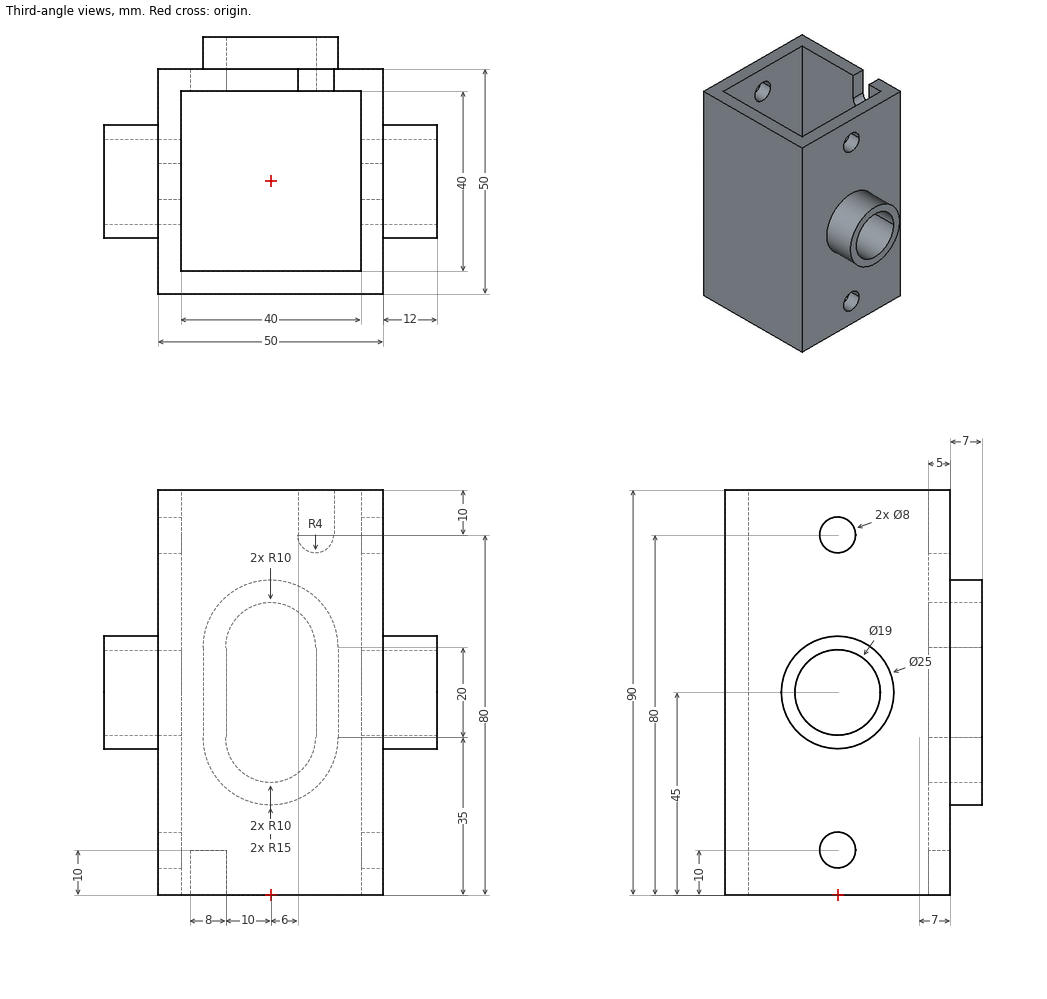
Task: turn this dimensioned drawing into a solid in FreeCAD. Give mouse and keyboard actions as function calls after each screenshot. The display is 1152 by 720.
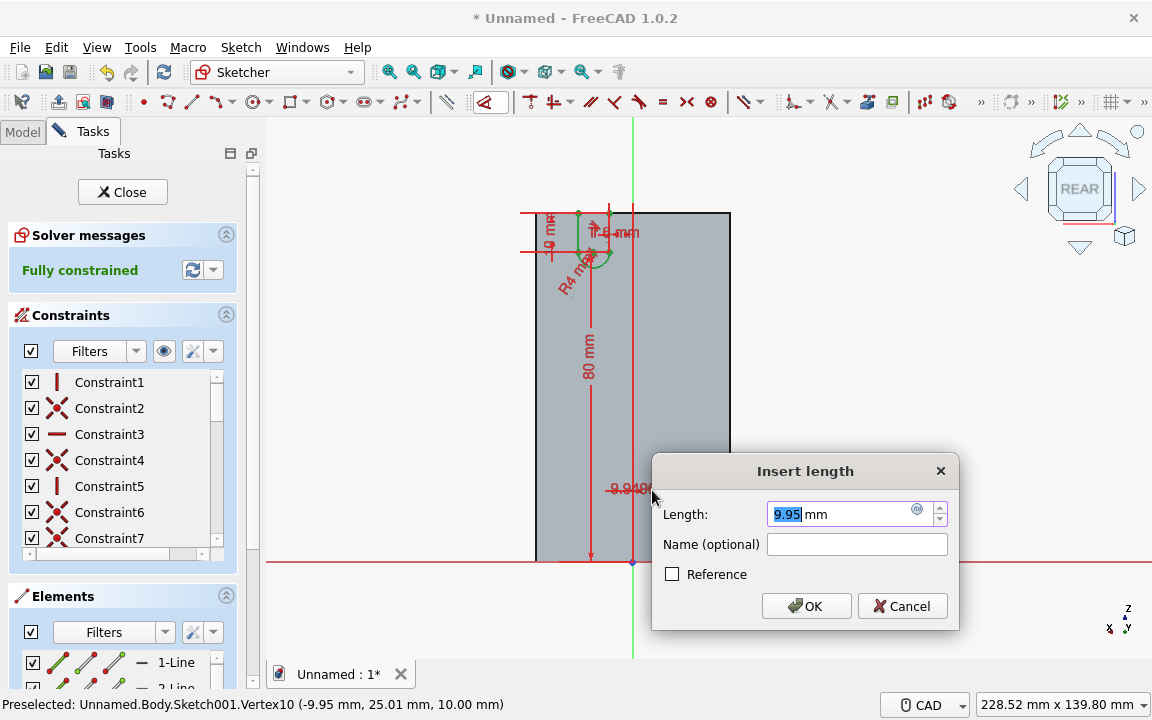
text(10)
key(Return)
key(Escape)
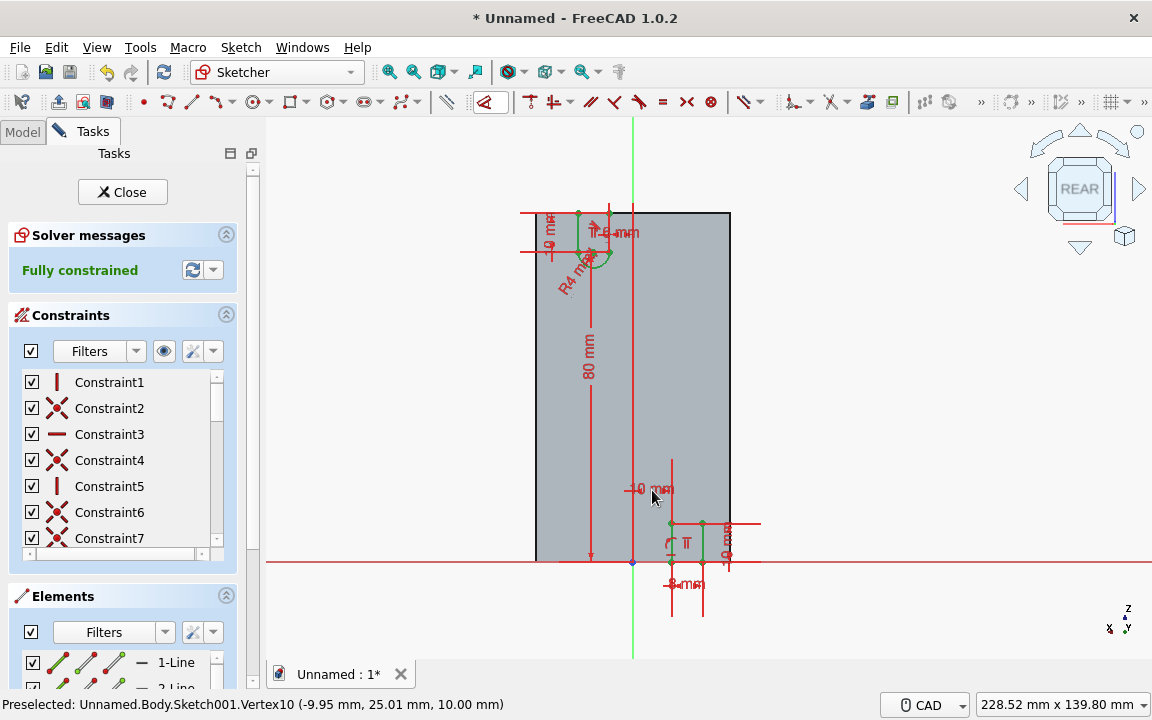
click(123, 192)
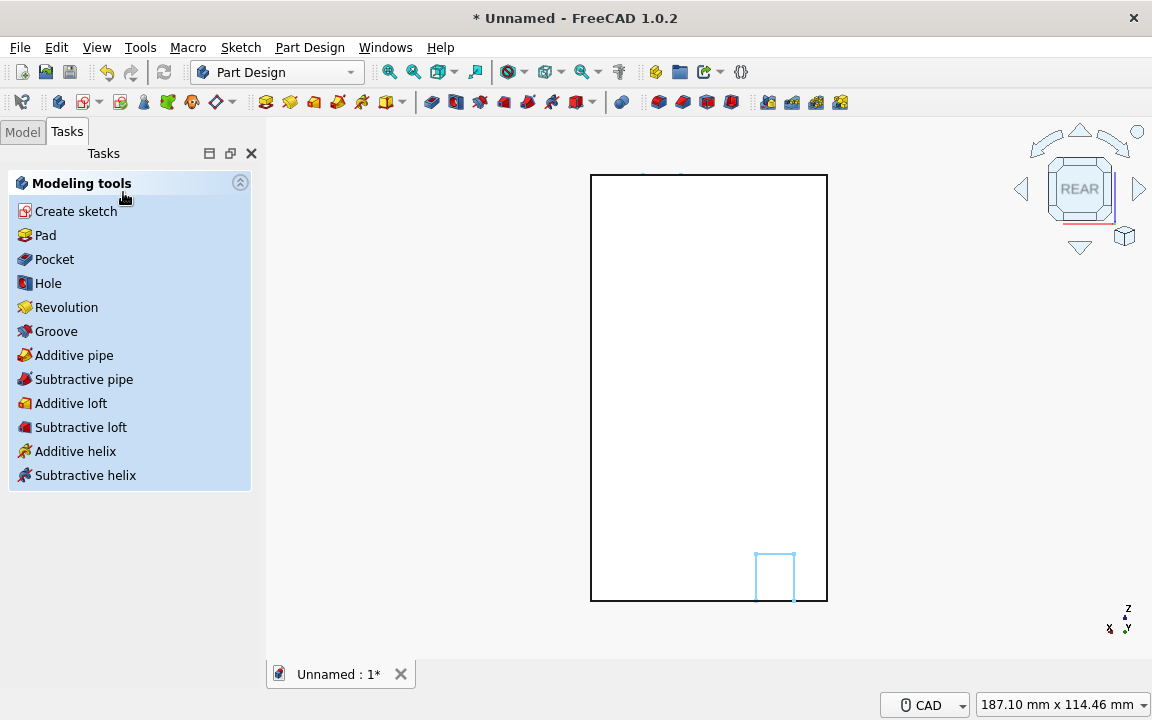
click(432, 102)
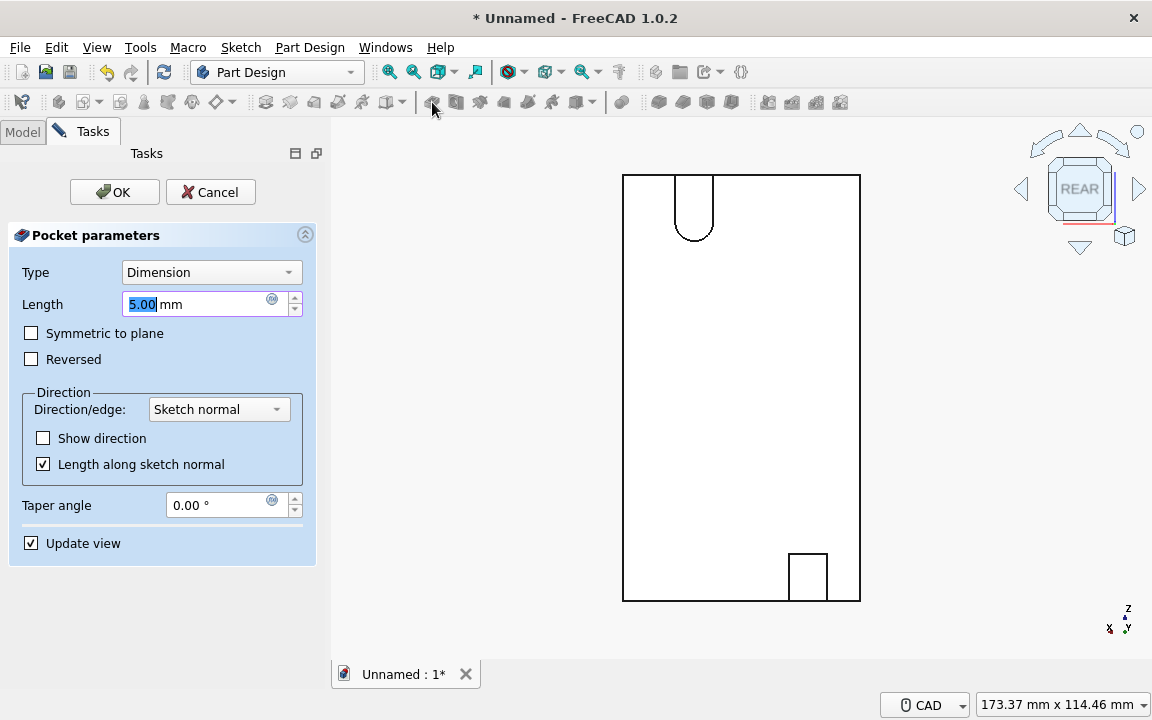
text(5)
key(Tab)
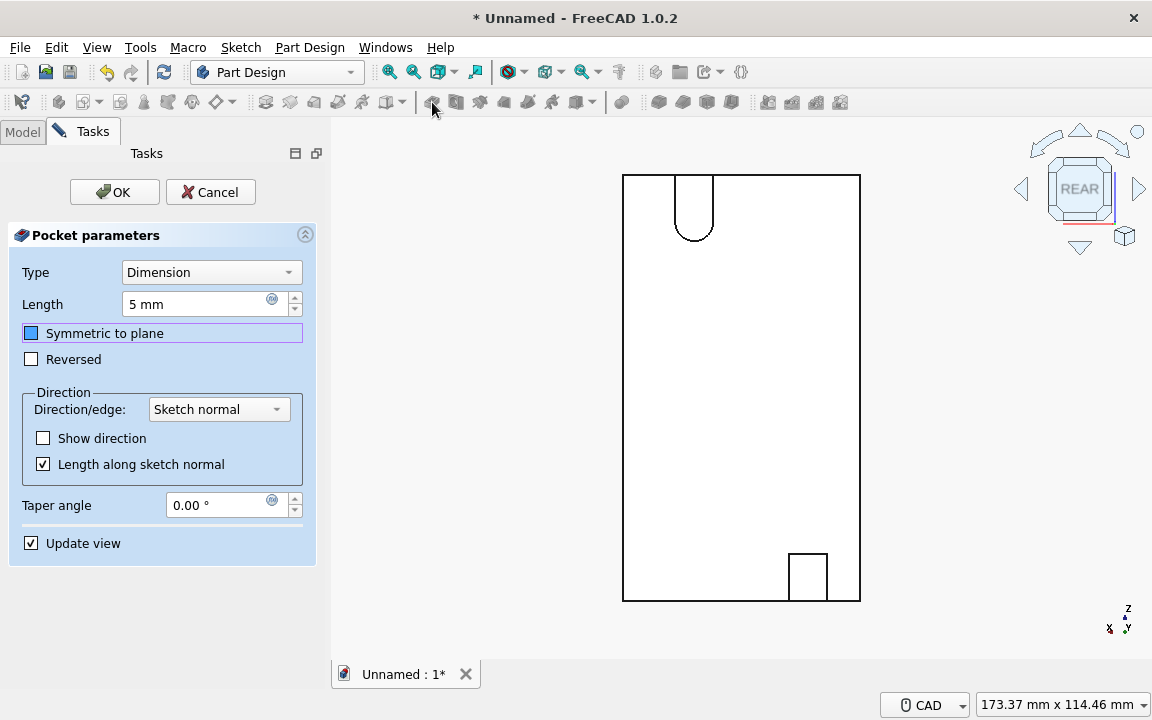
click(115, 192)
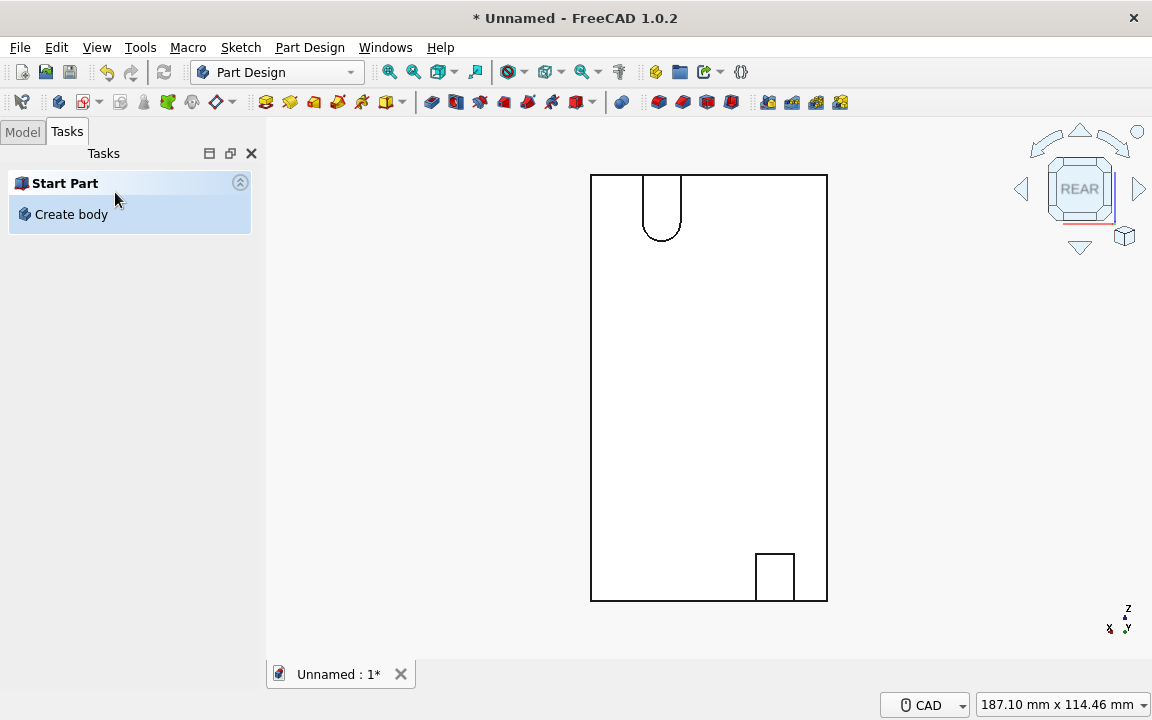
click(709, 387)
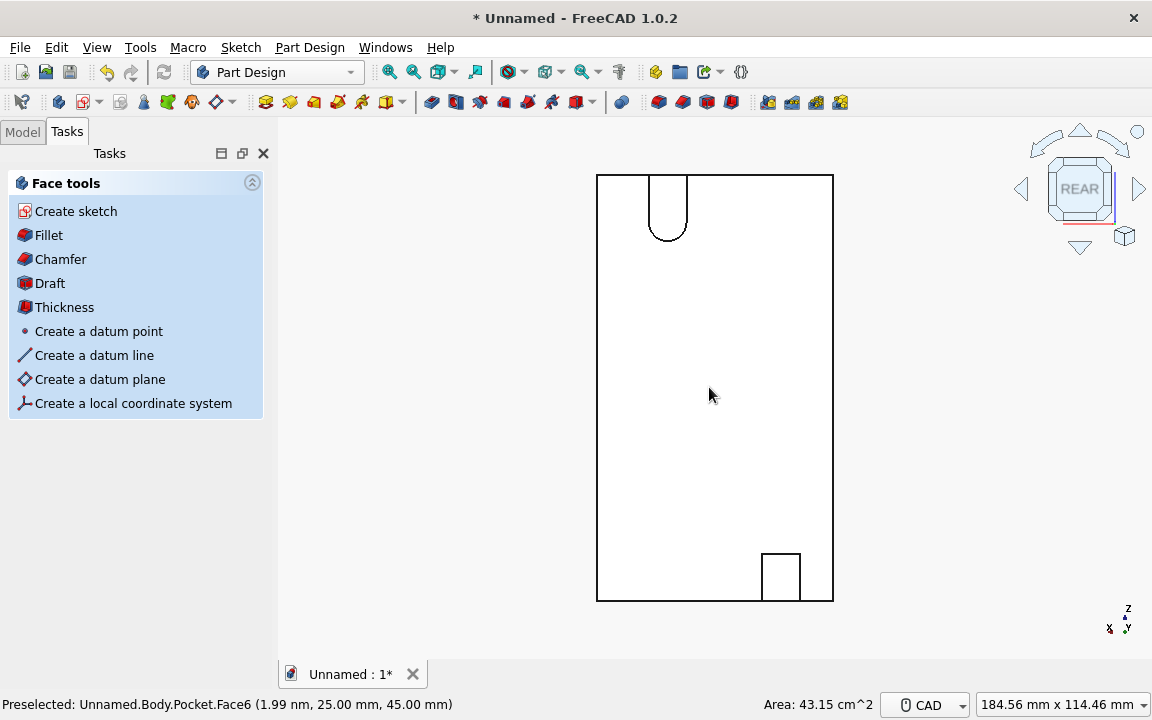
click(84, 102)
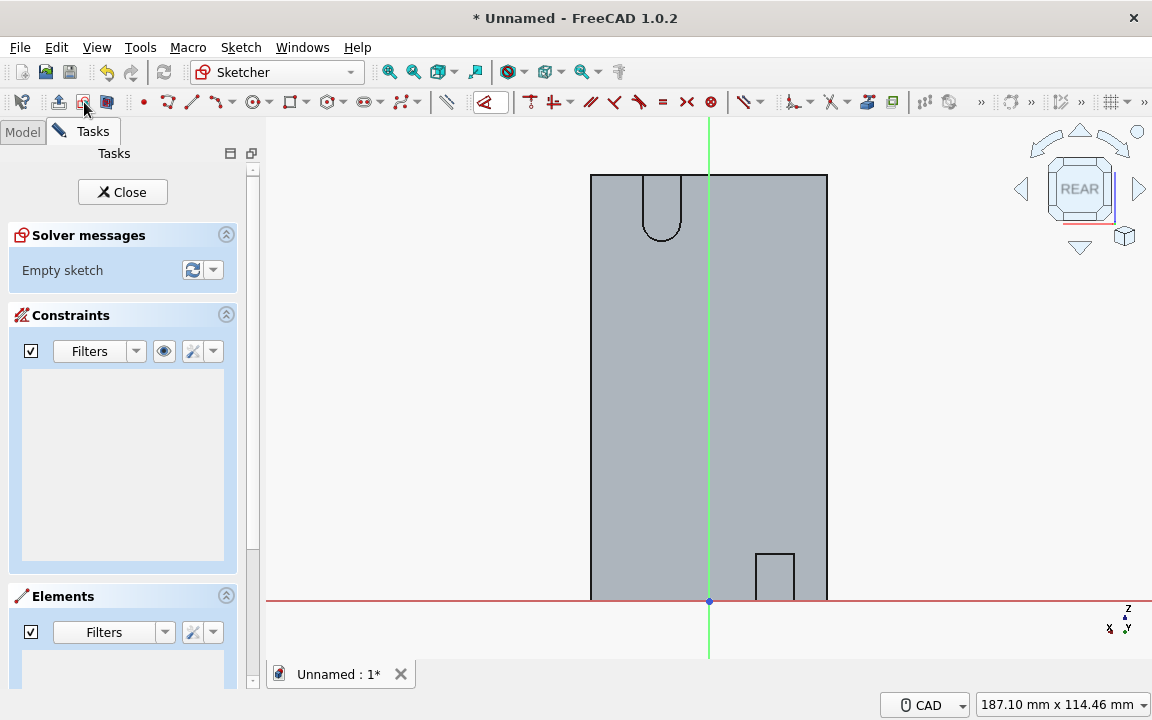
key(g)
key(s)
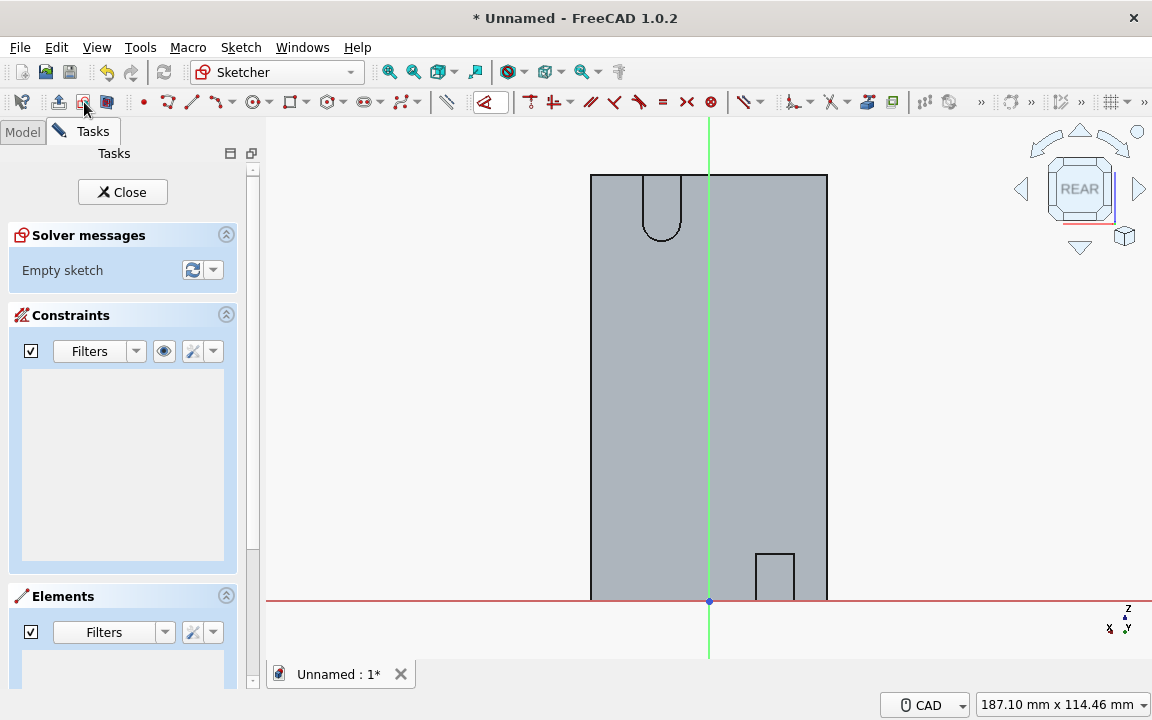
click(709, 435)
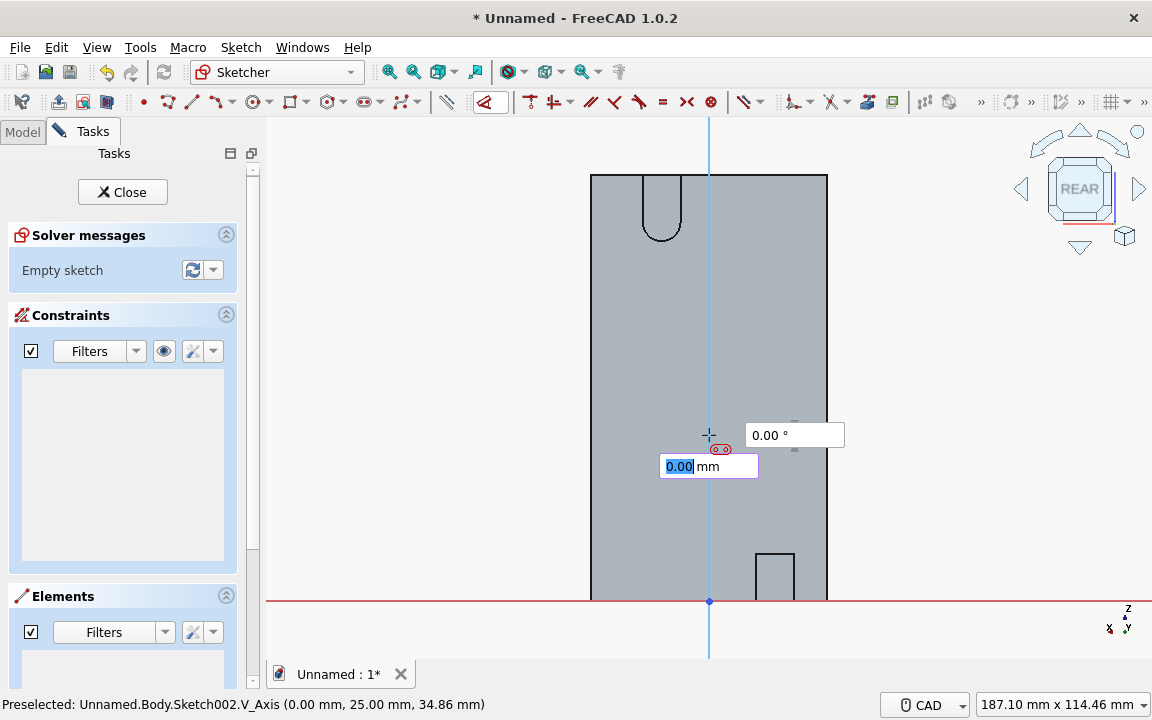
click(718, 341)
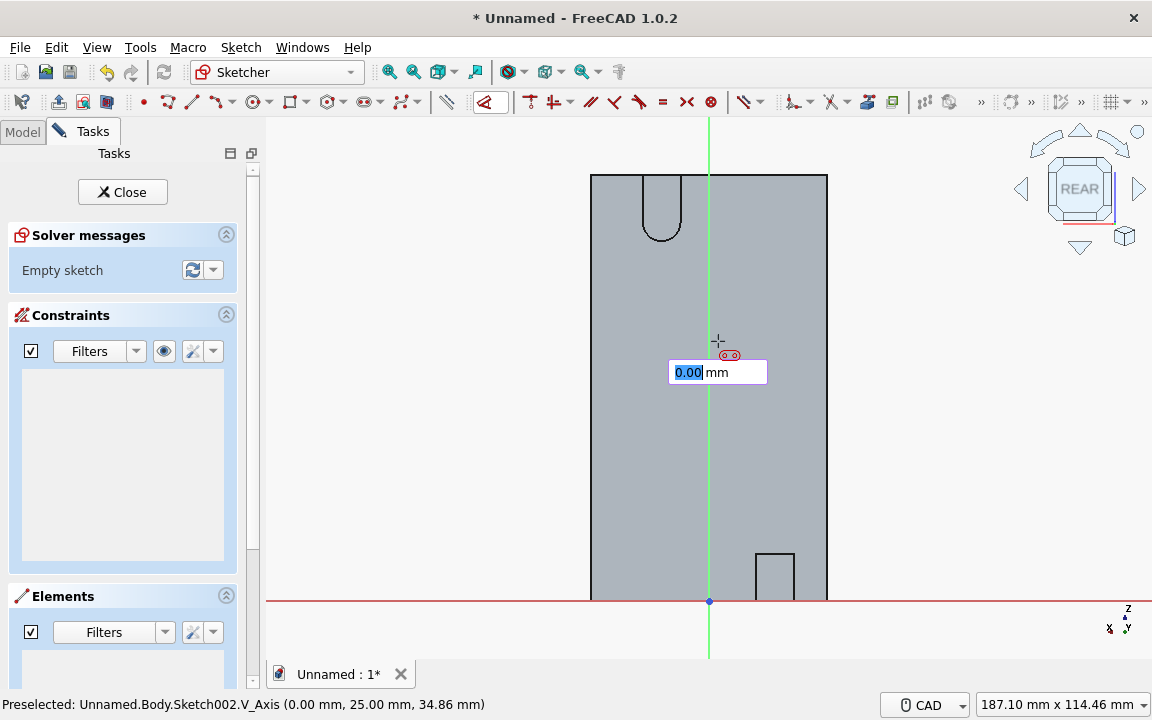
click(638, 388)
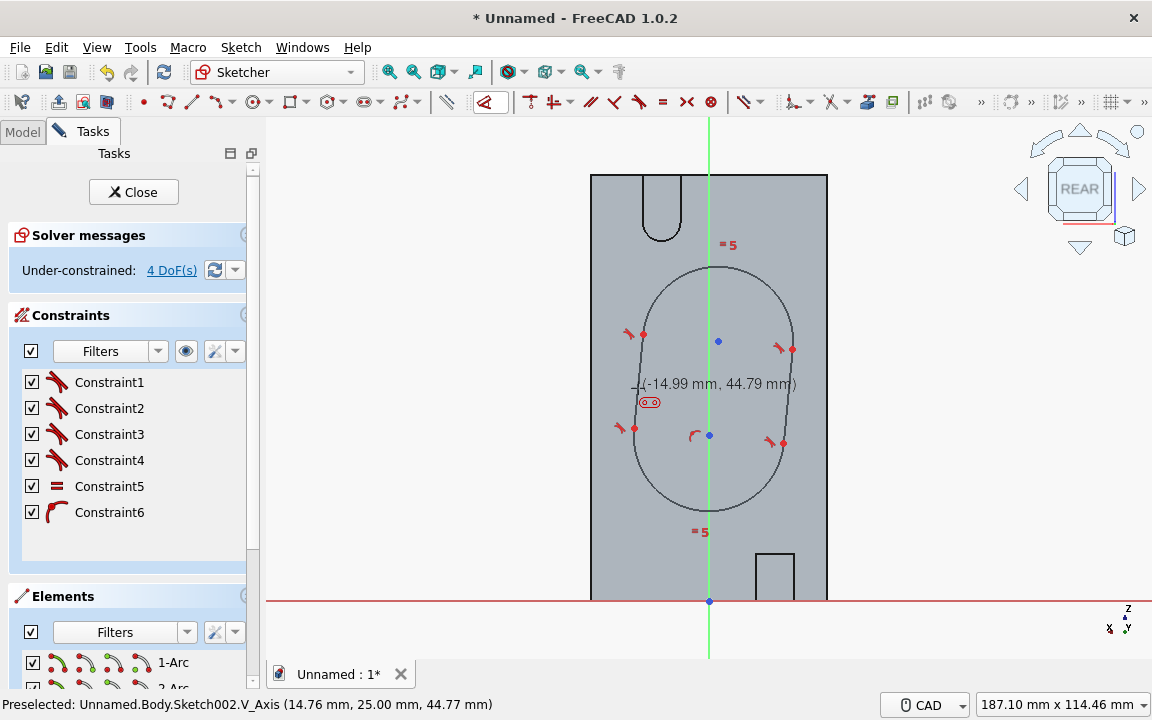
click(709, 436)